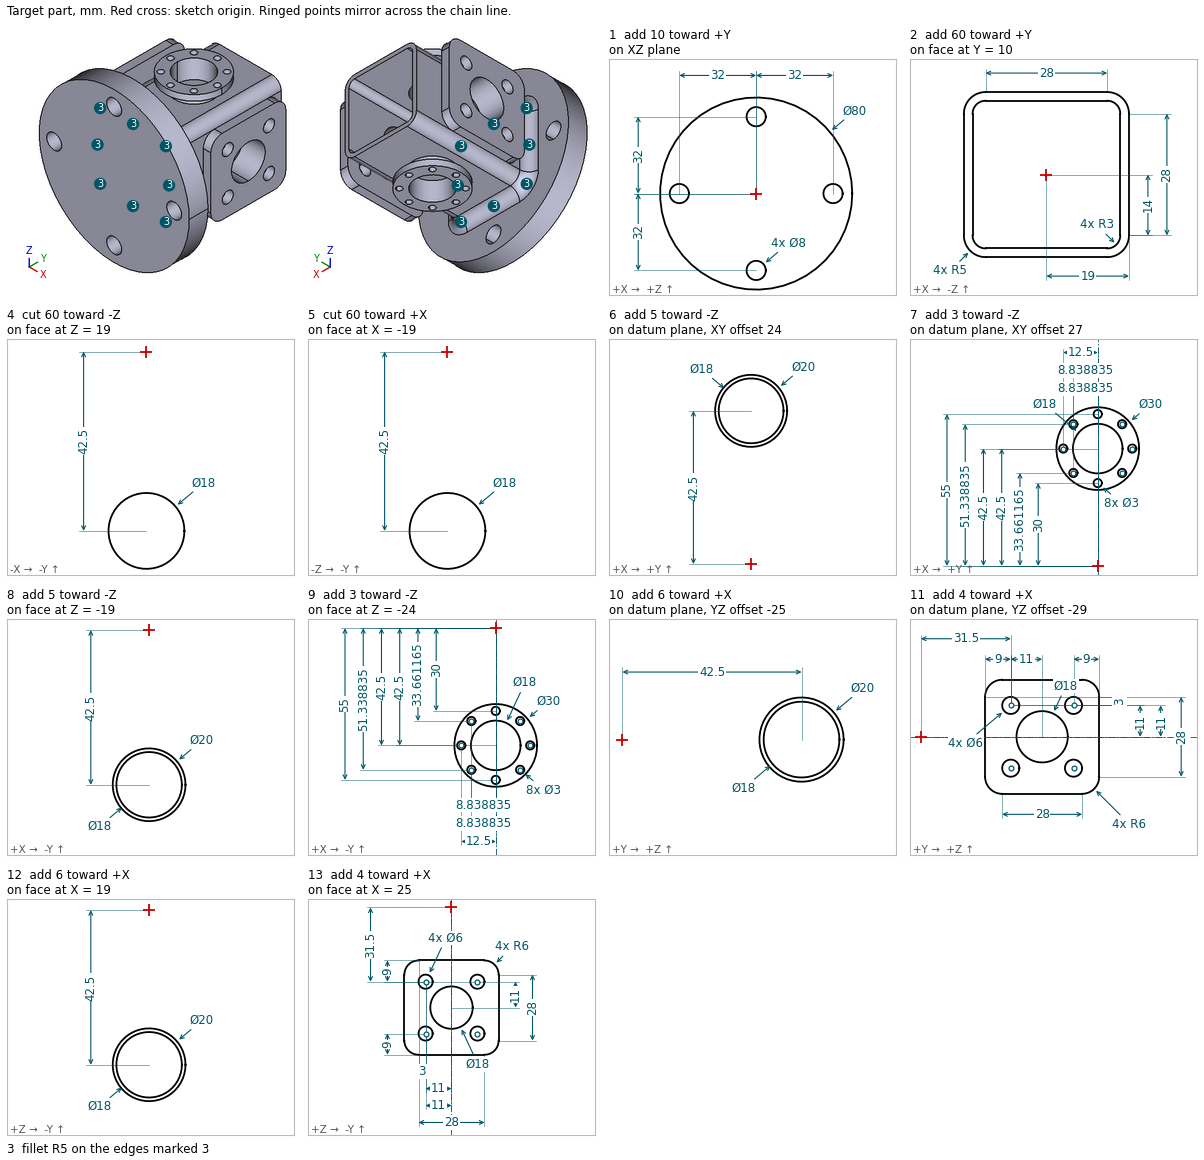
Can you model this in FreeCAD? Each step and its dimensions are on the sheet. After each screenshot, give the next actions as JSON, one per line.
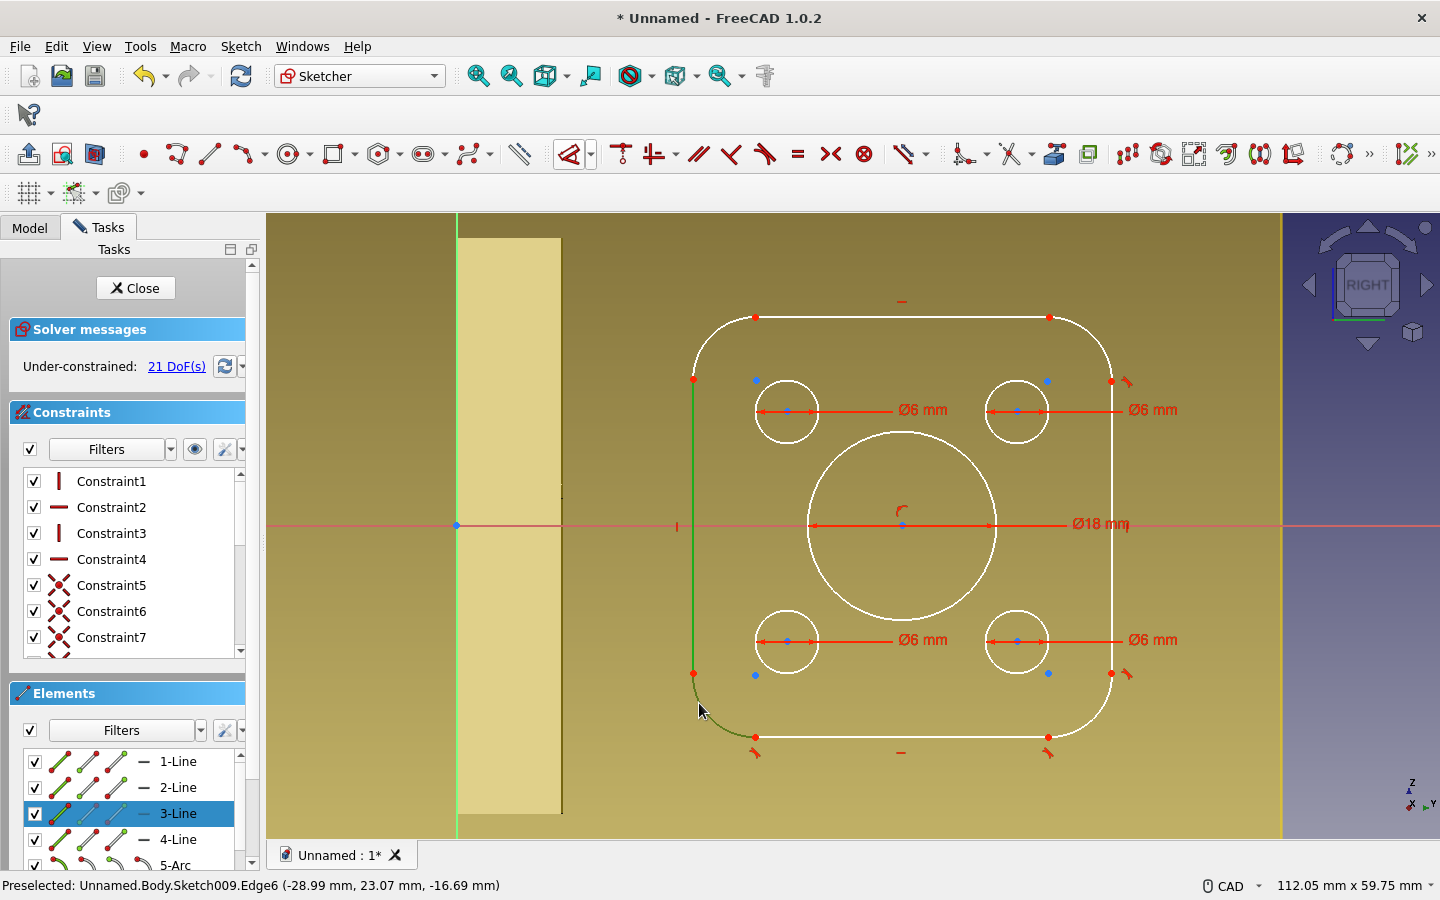
{"action": "key", "text": "t"}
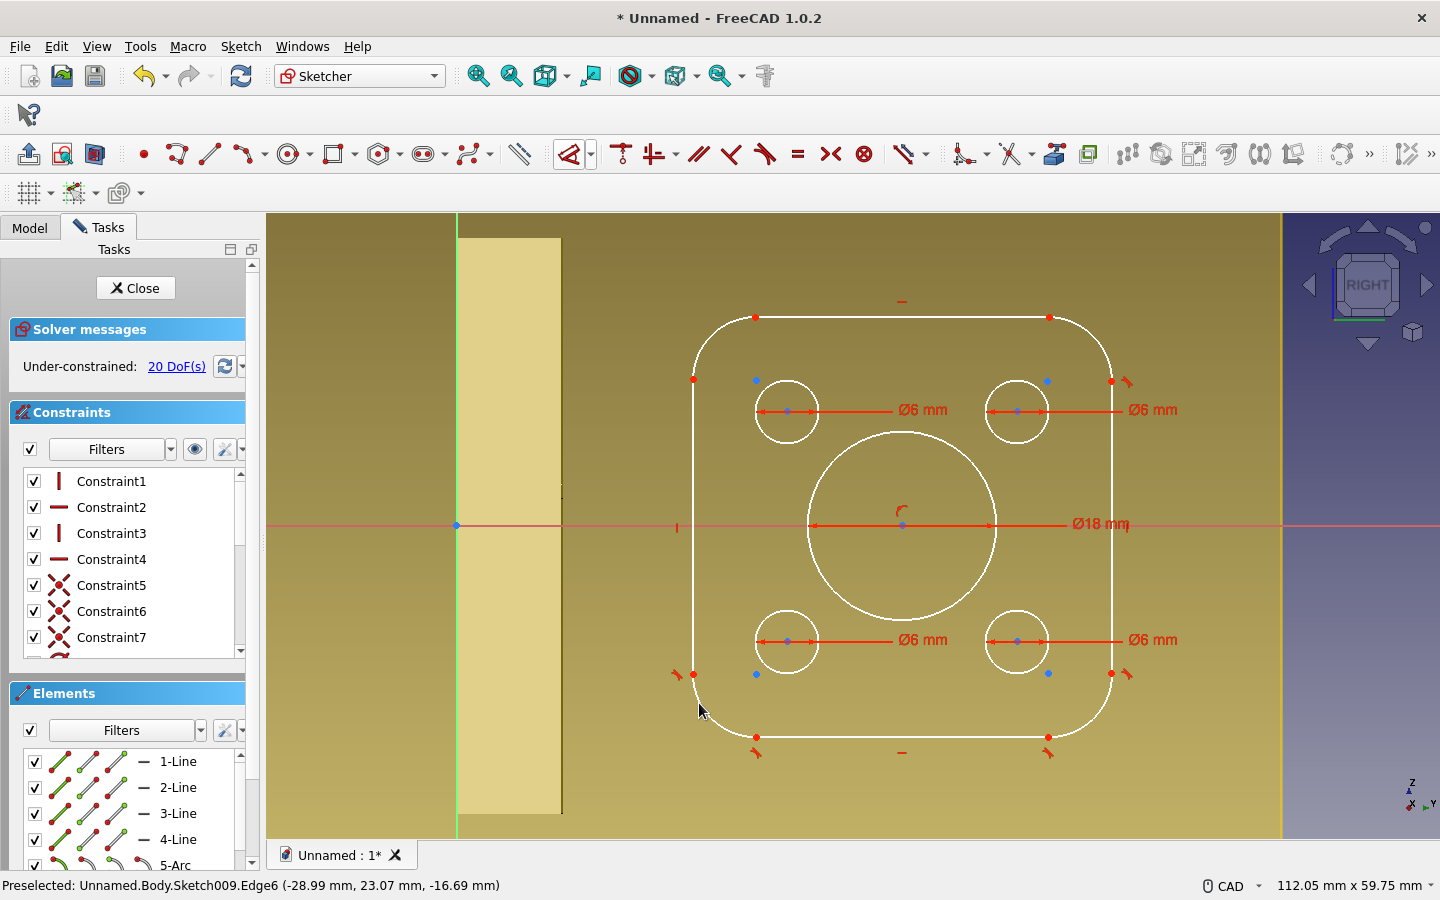
{"action": "left_click", "coordinate": [693, 586]}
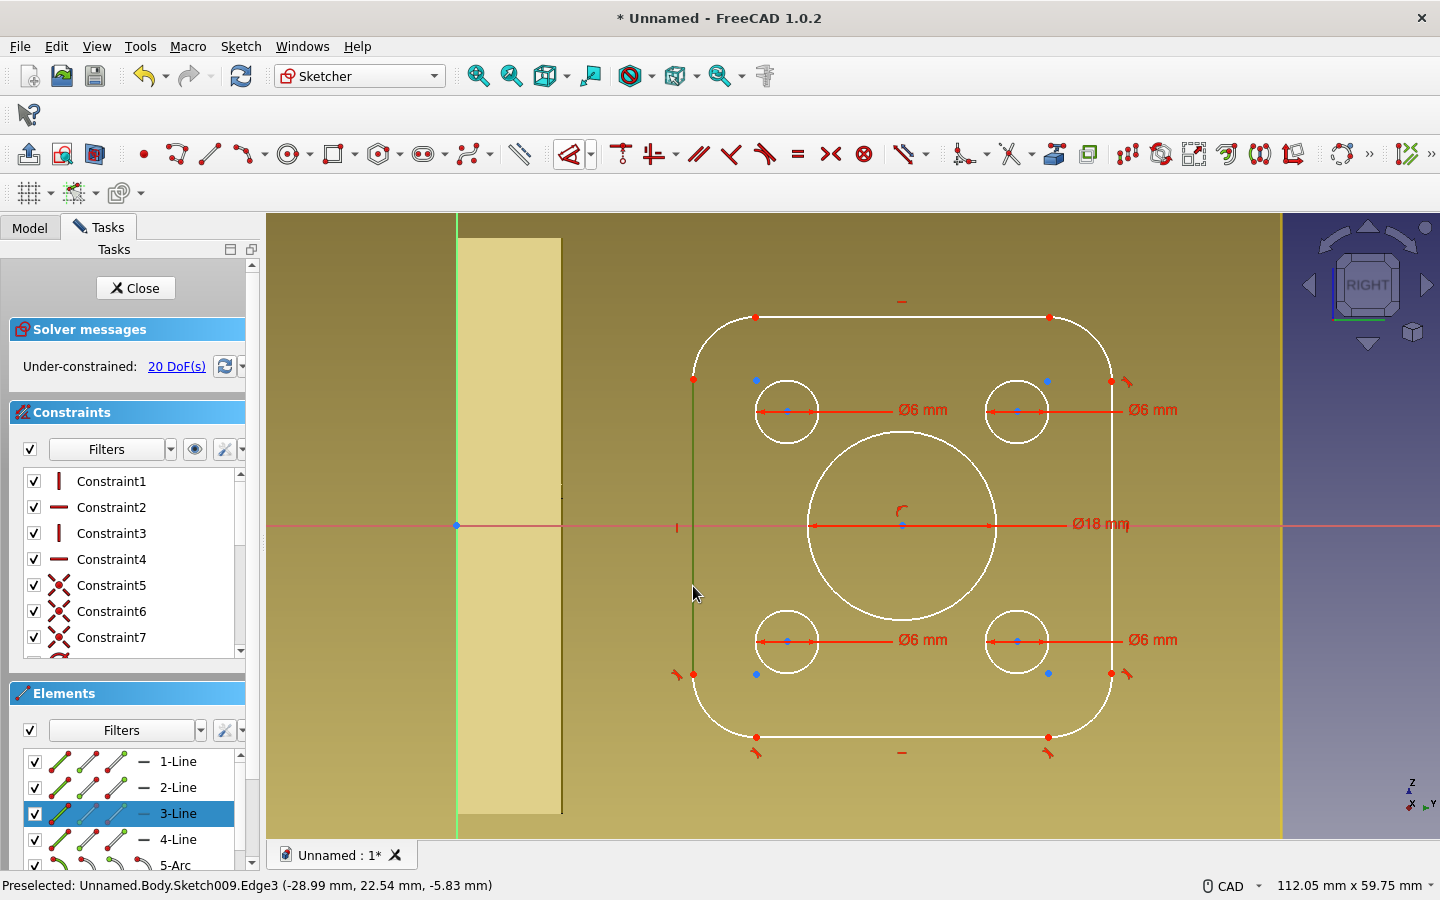
{"action": "left_click", "coordinate": [727, 324]}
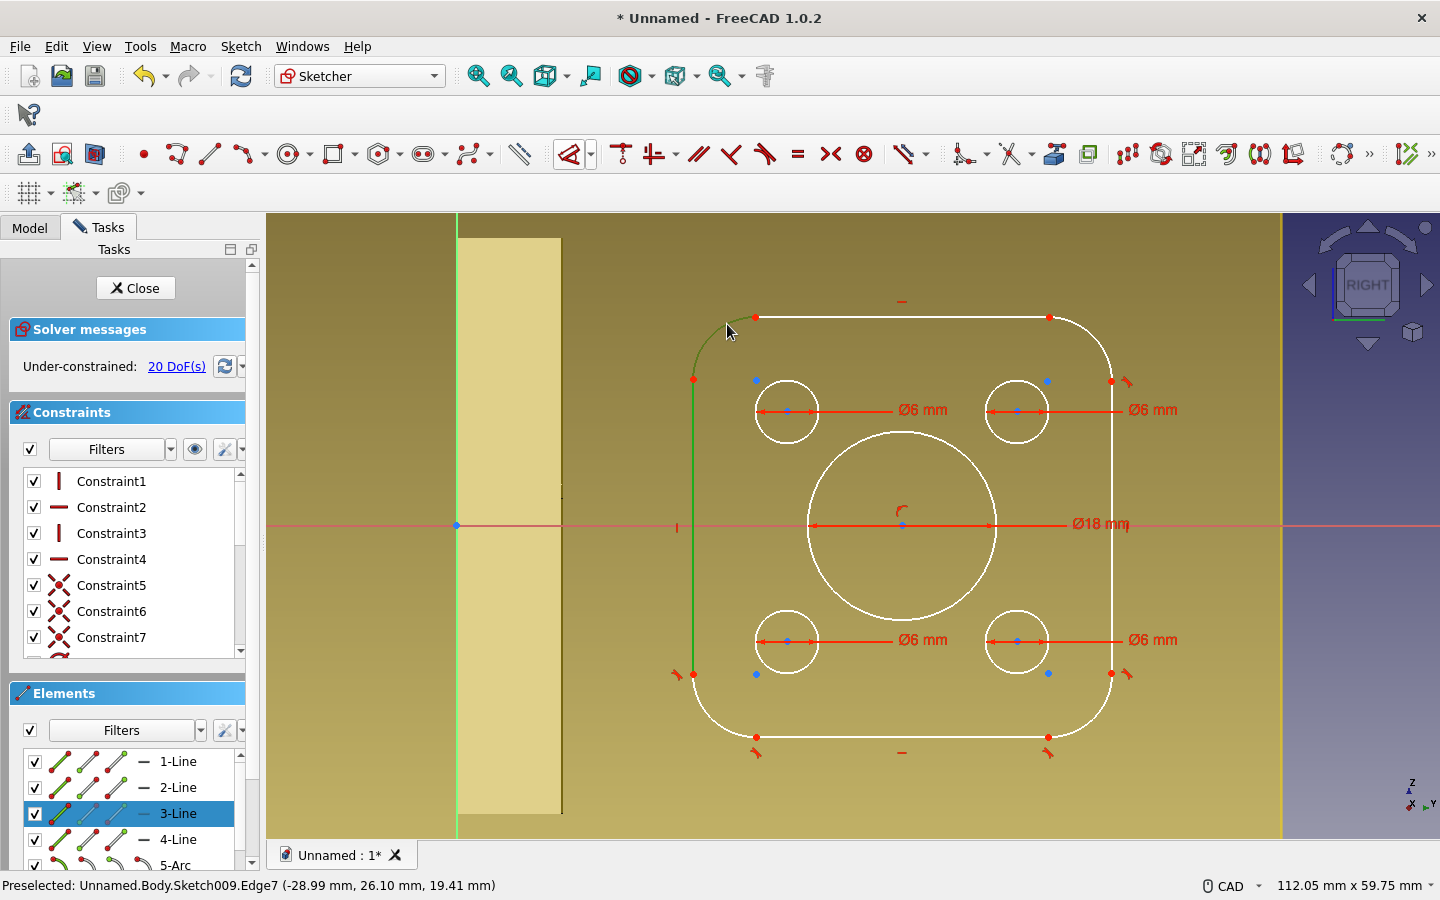
{"action": "key", "text": "t"}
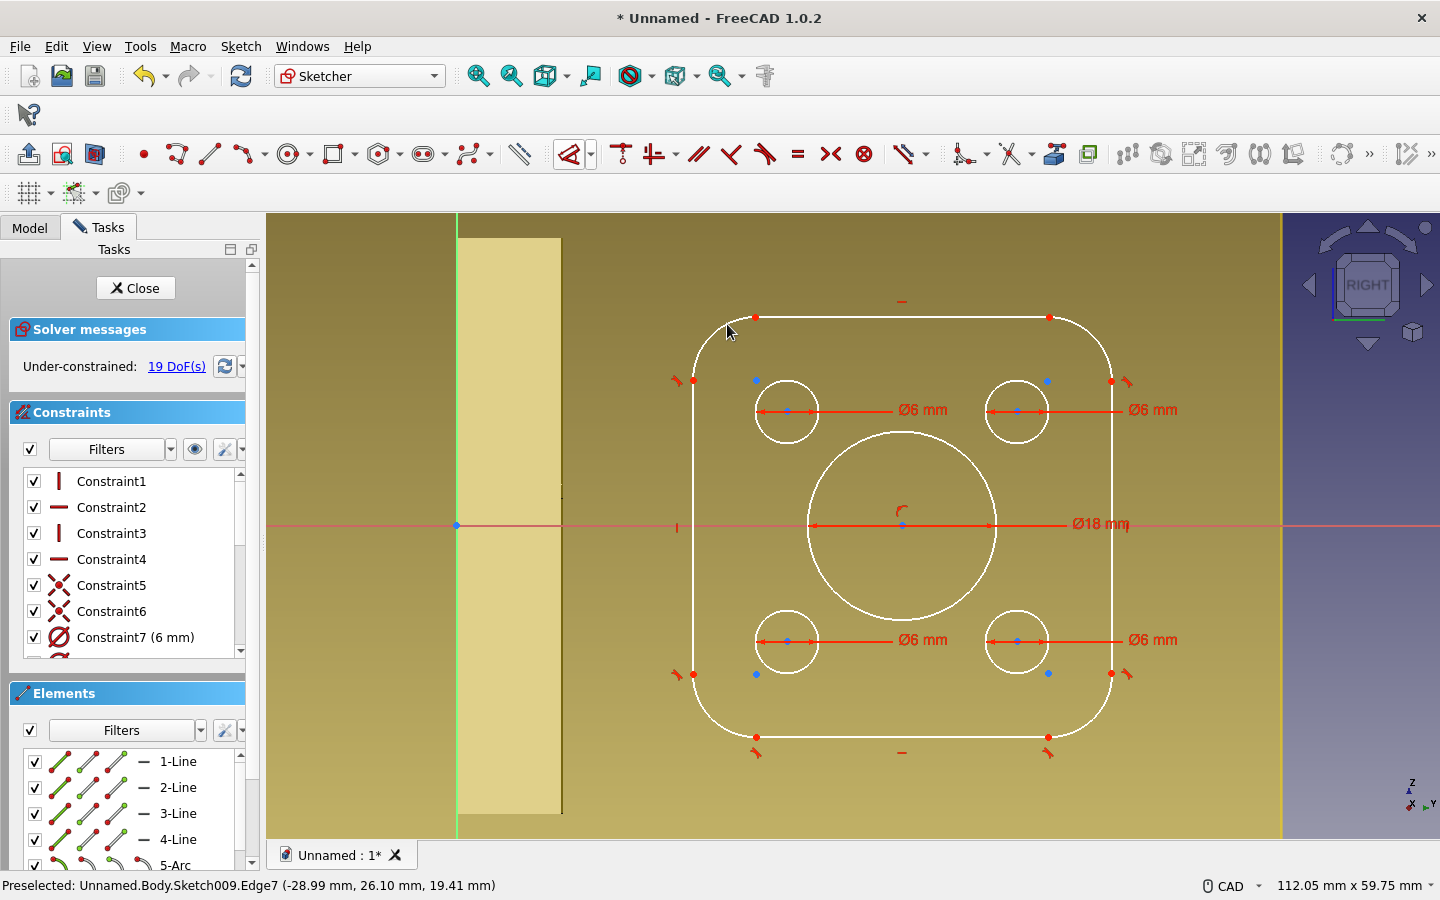
{"action": "left_click", "coordinate": [843, 317]}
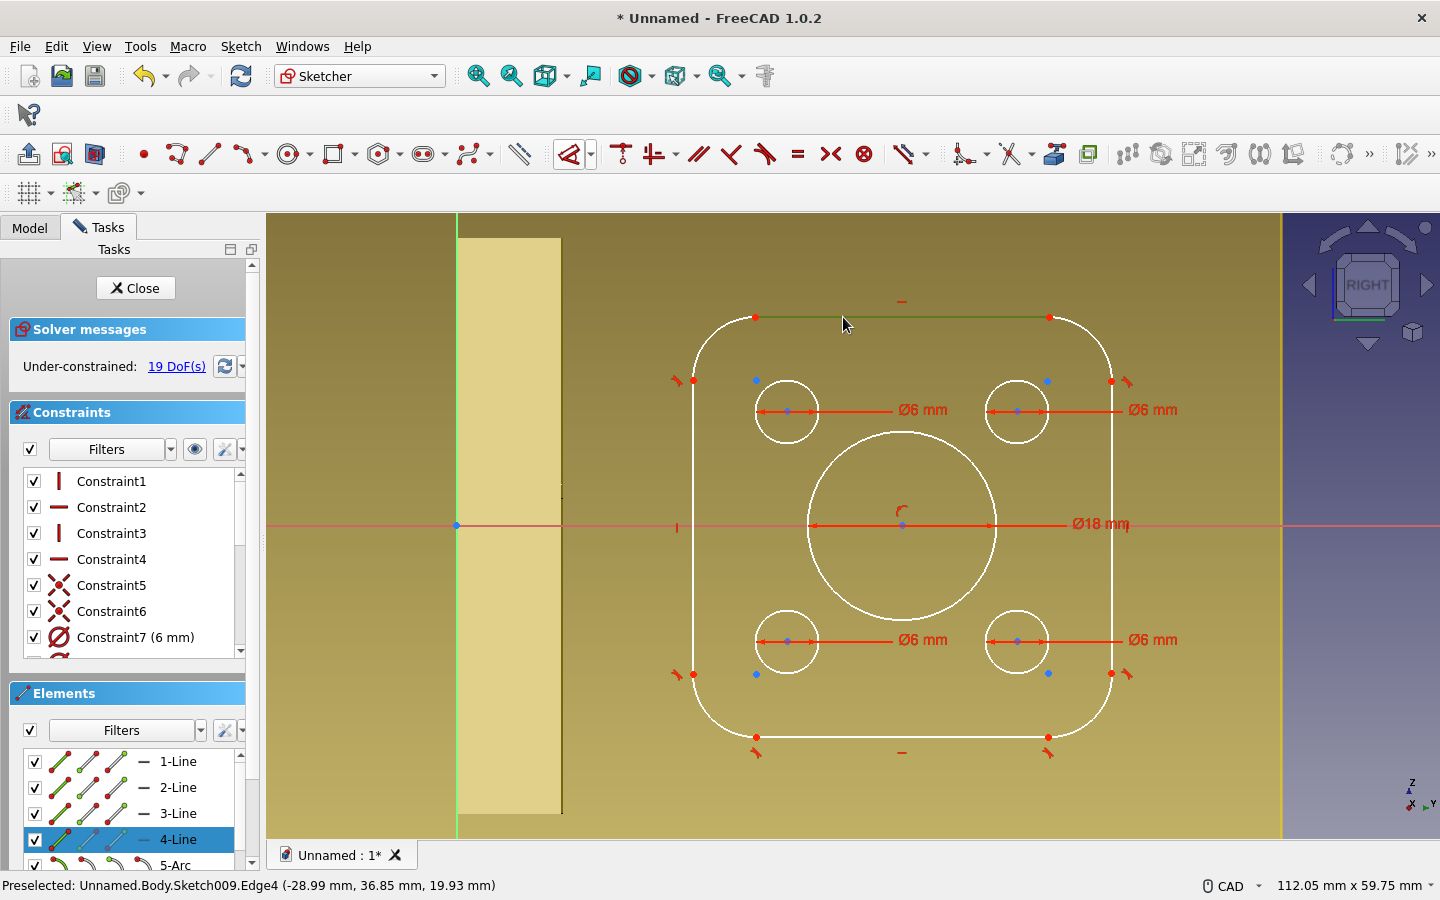
{"action": "left_click", "coordinate": [727, 324]}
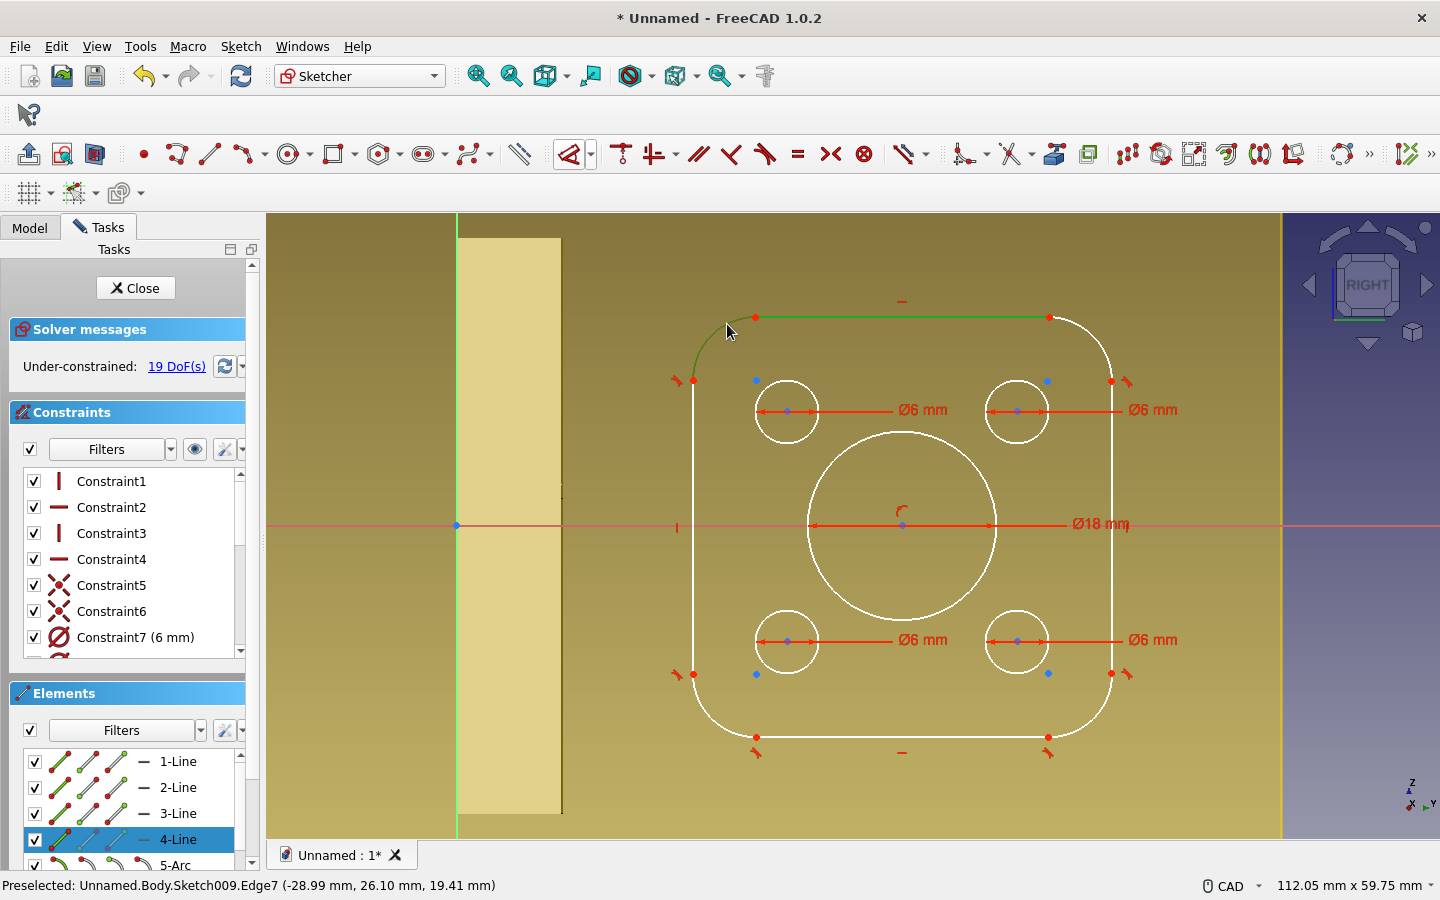
{"action": "key", "text": "t"}